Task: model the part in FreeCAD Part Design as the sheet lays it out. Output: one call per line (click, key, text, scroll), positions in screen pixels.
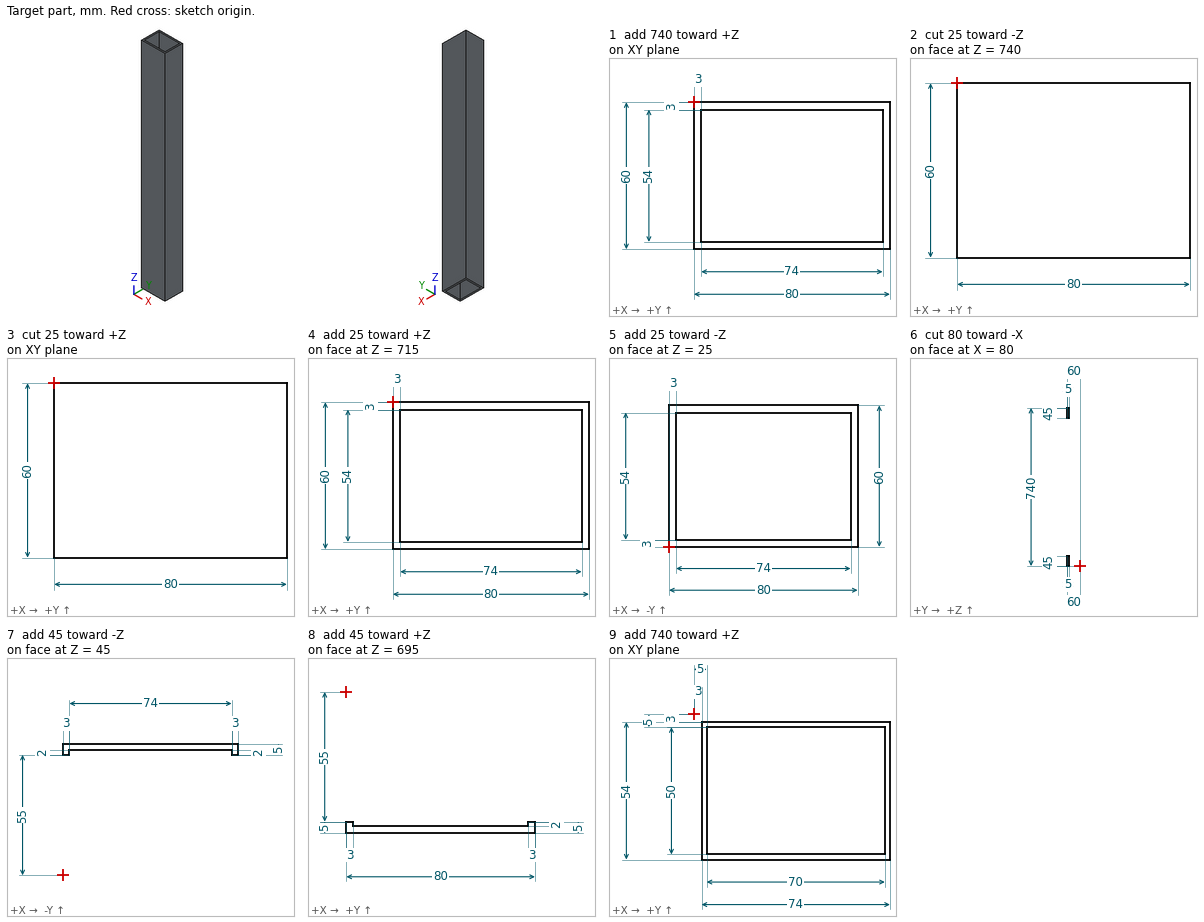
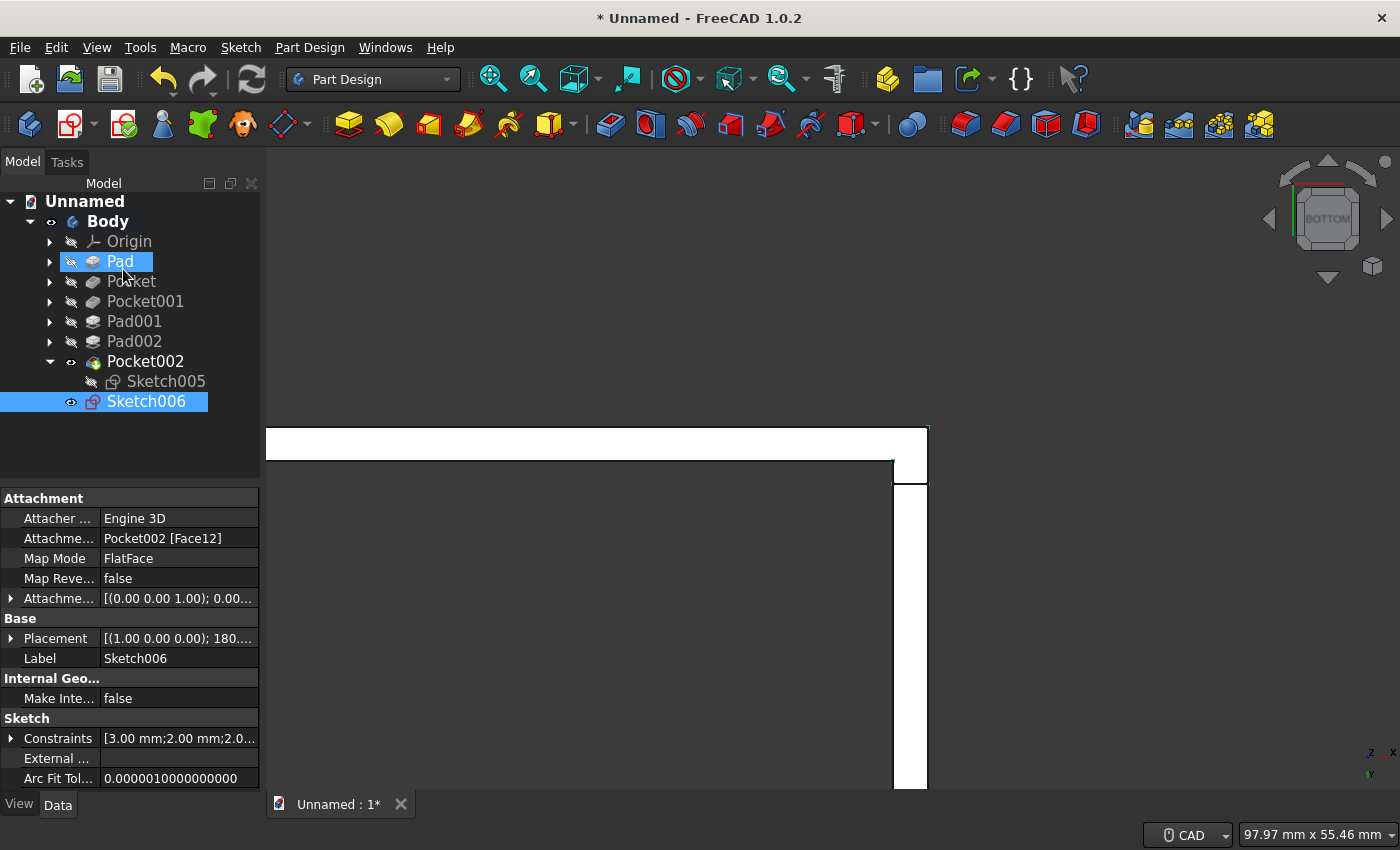
click(350, 124)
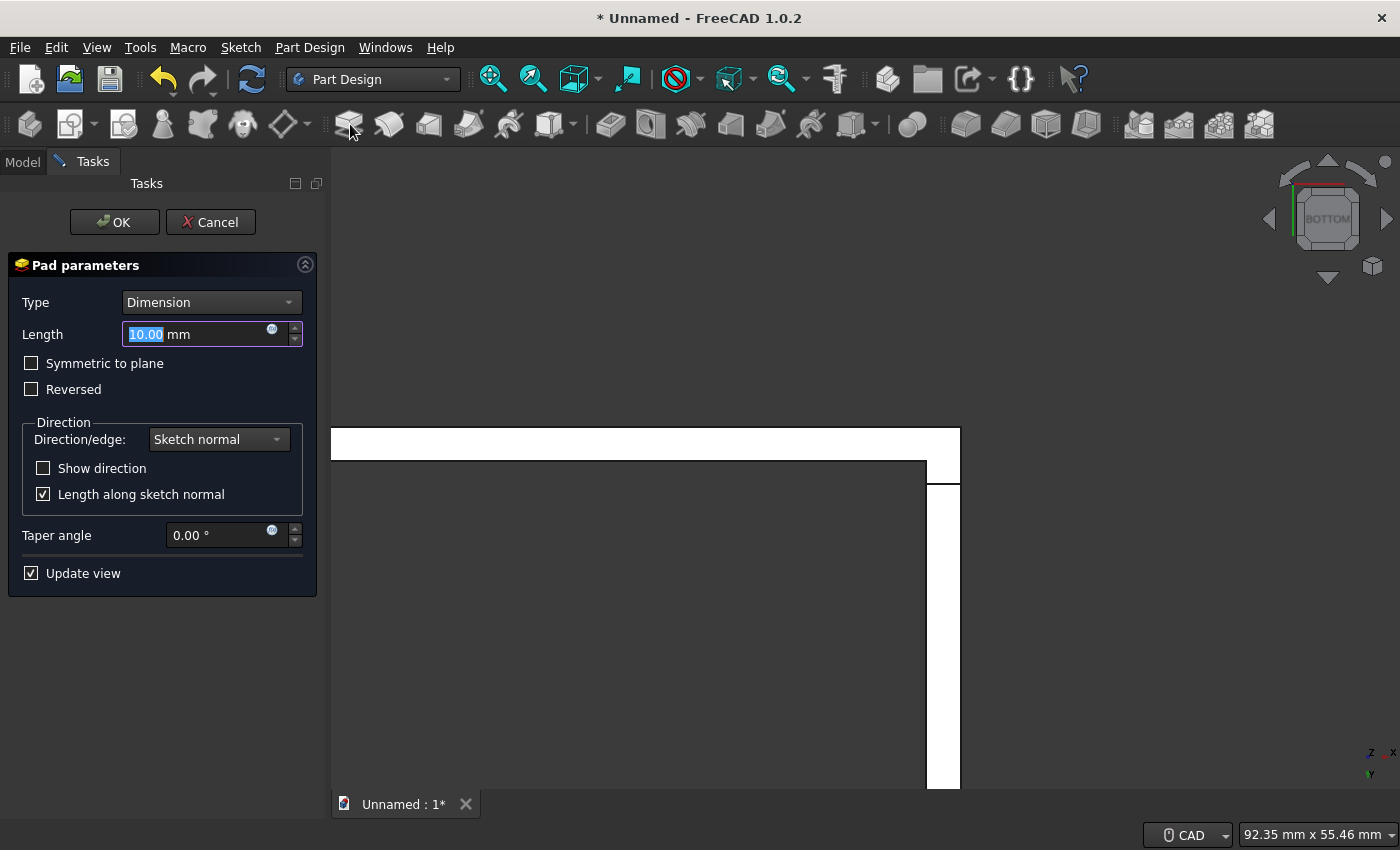
text(45)
key(Tab)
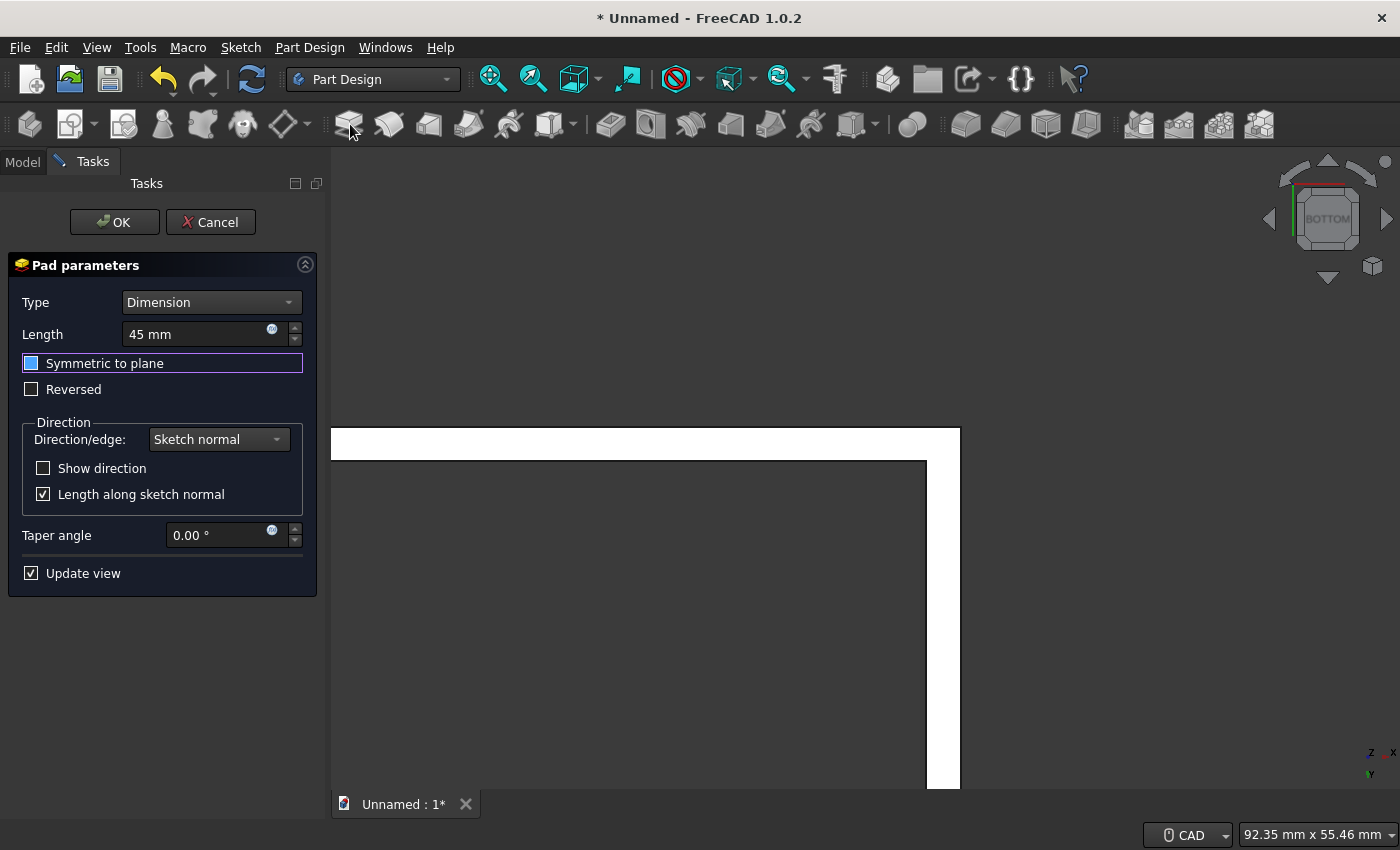
click(115, 222)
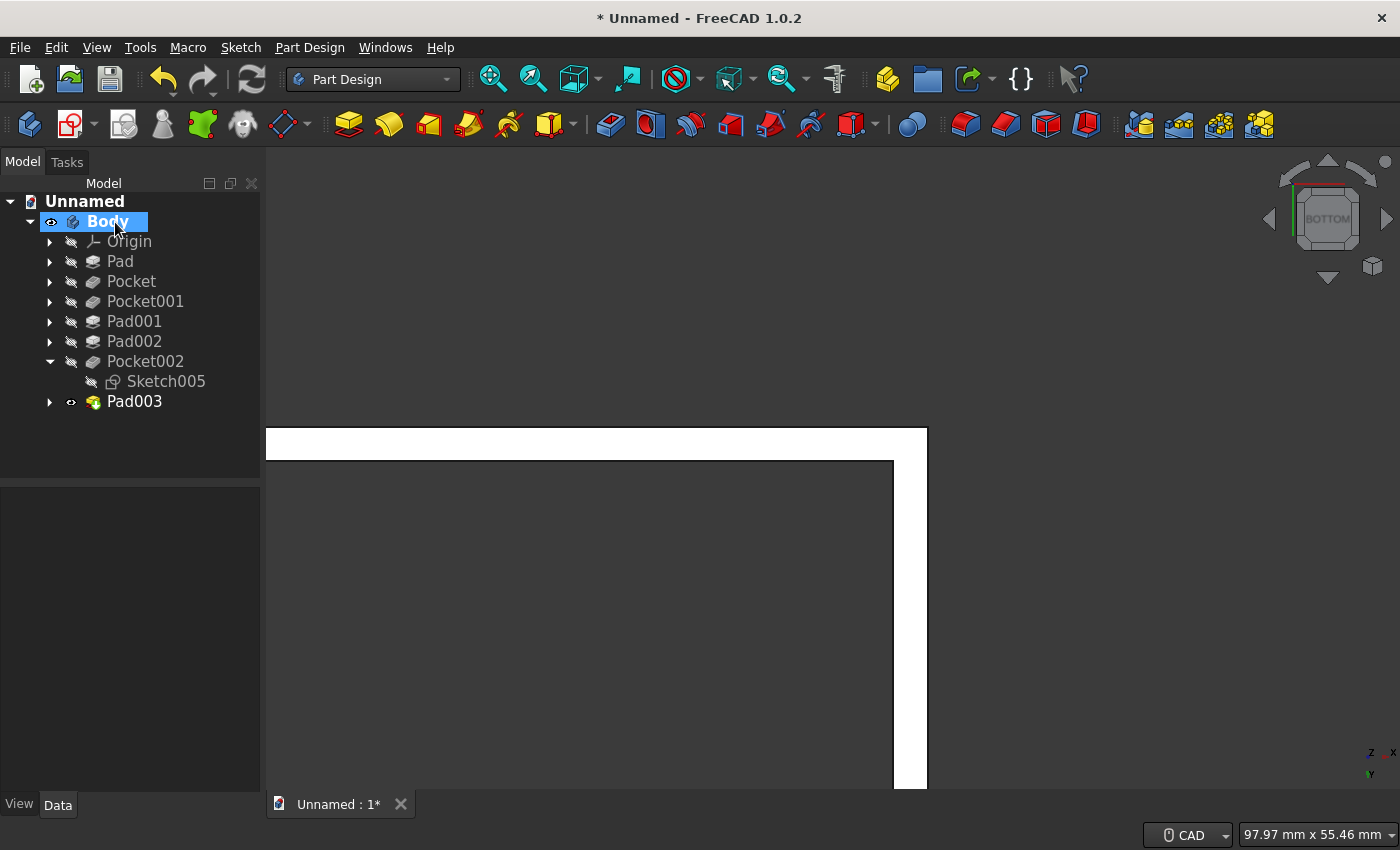
key(v)
key(f)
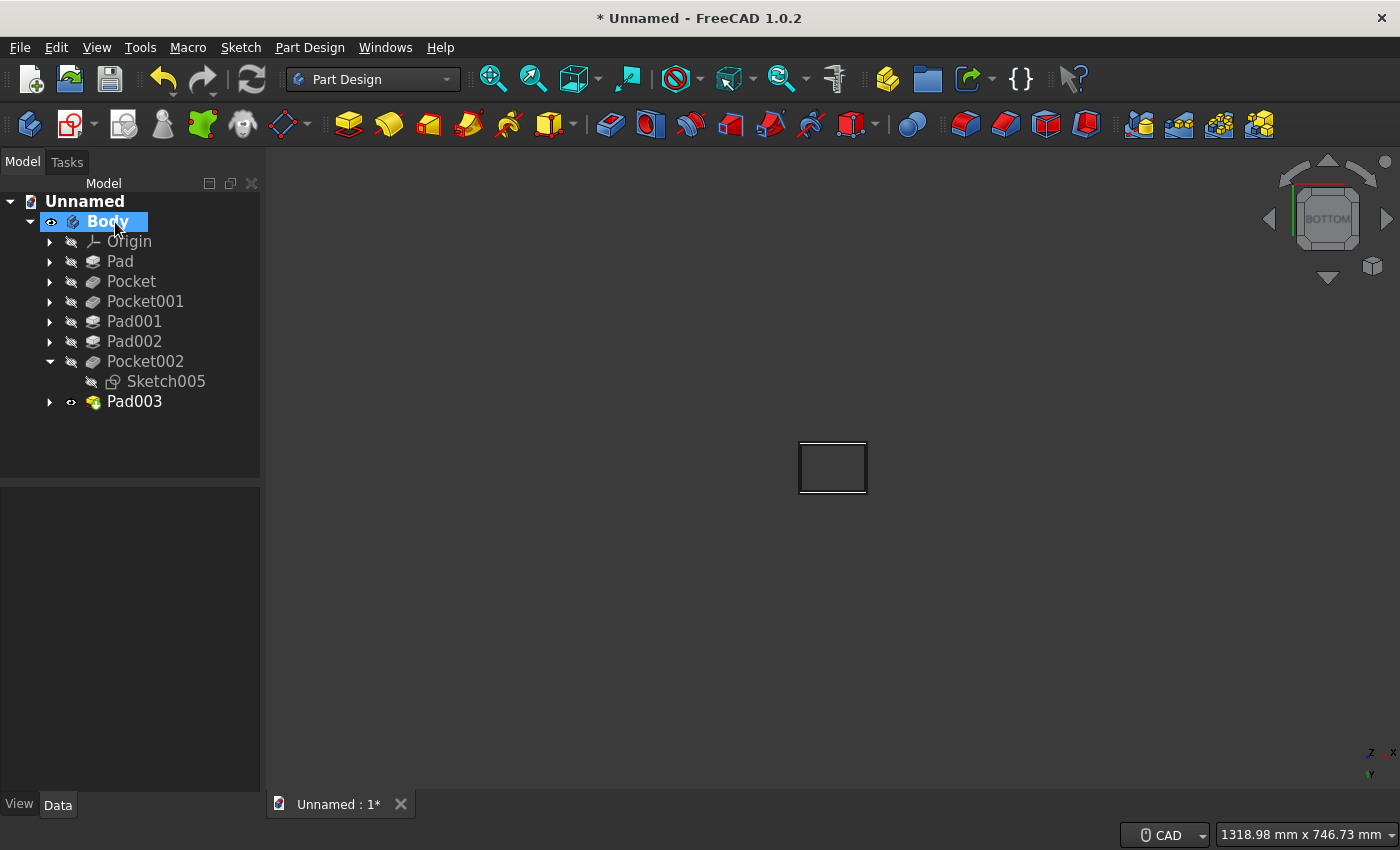
key(0)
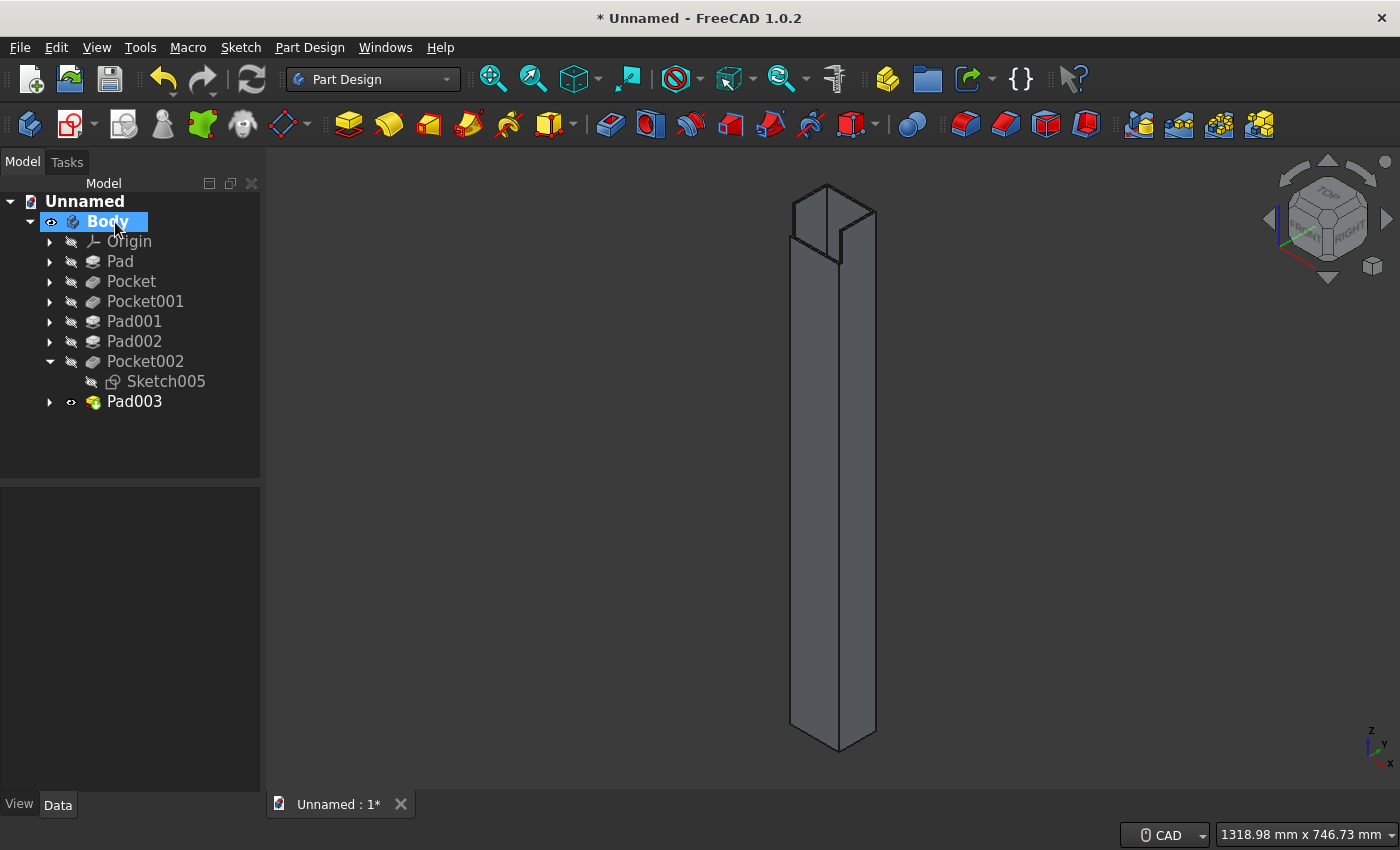
scroll(837, 261, up, 13)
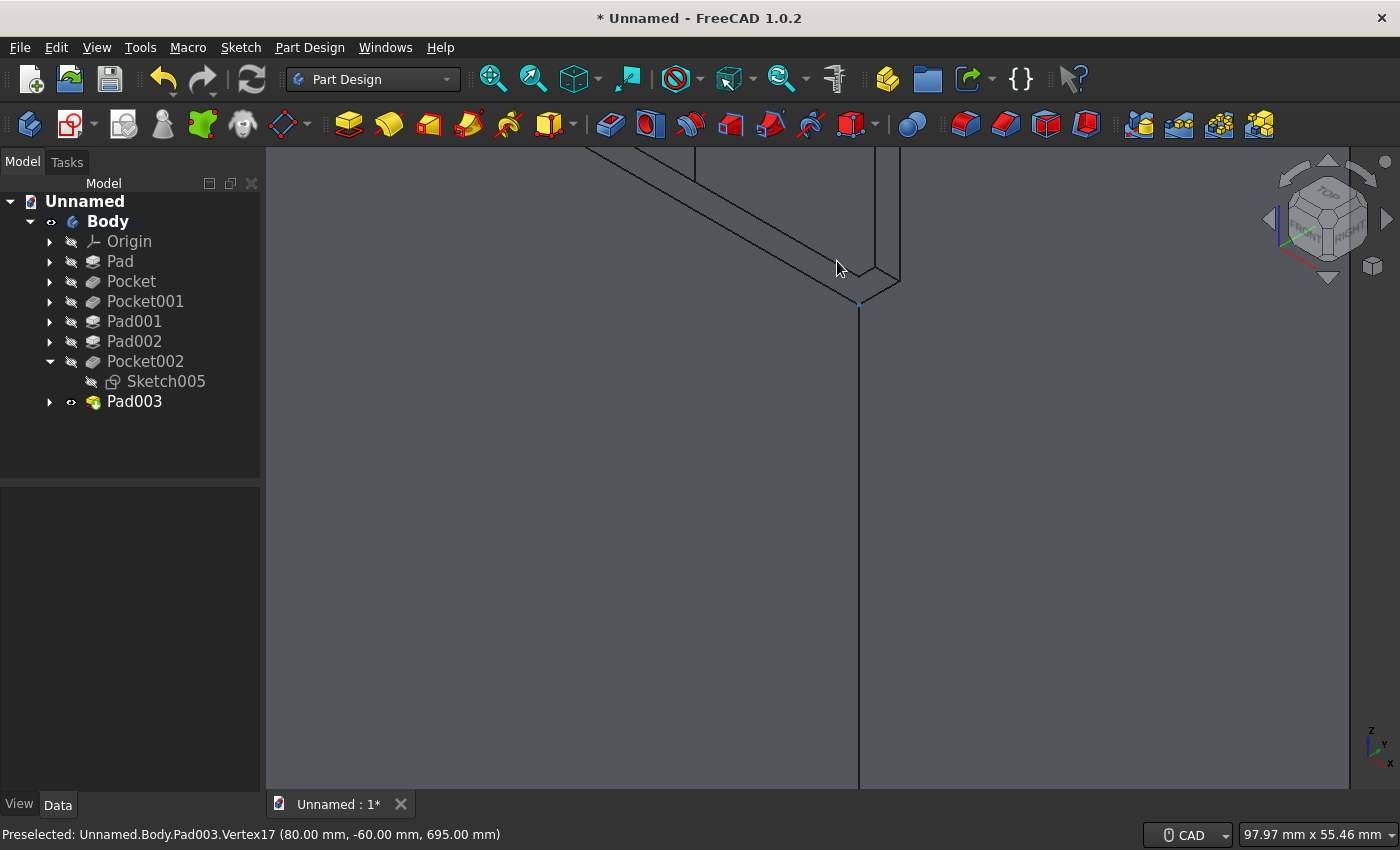
click(827, 268)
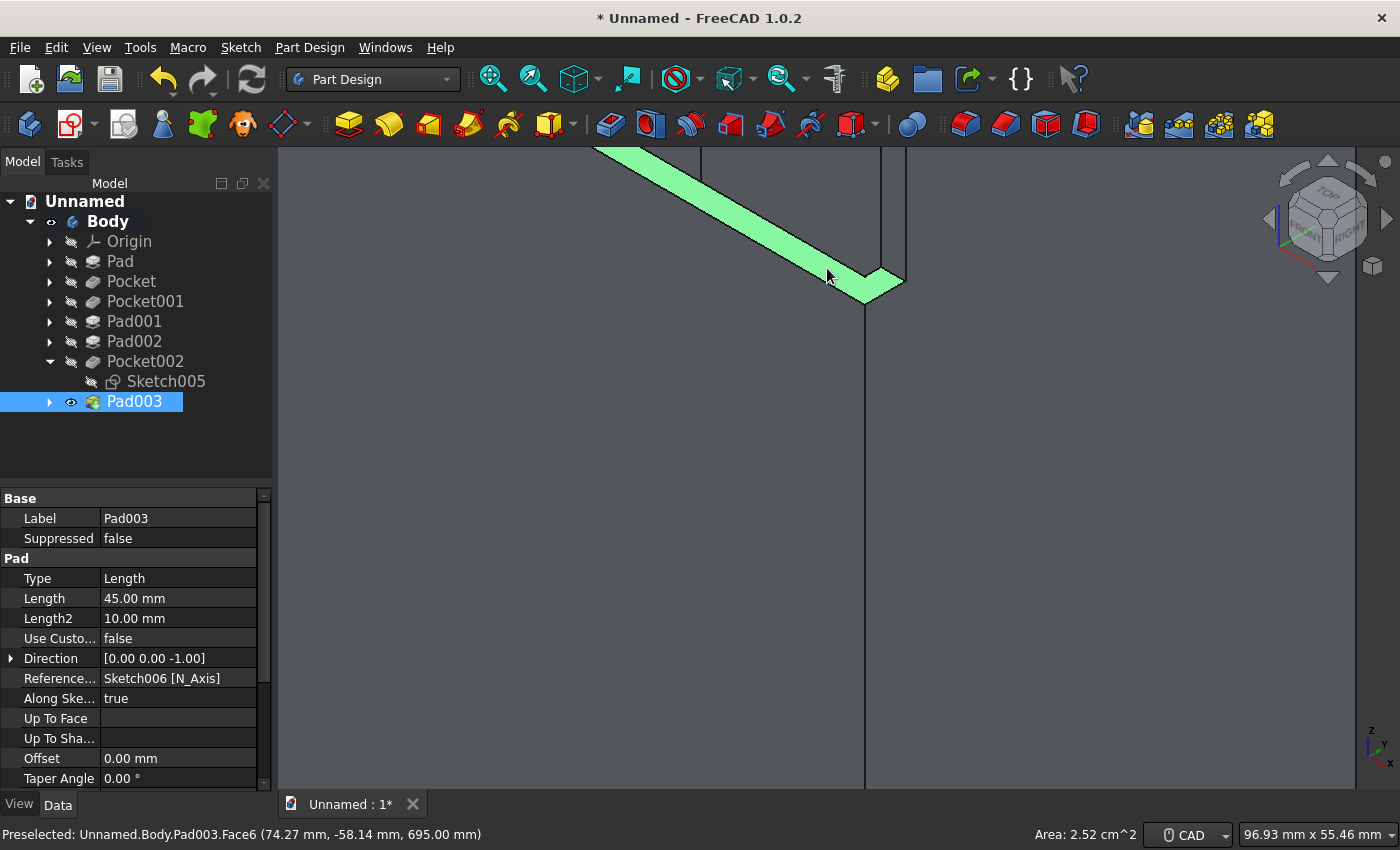
click(70, 124)